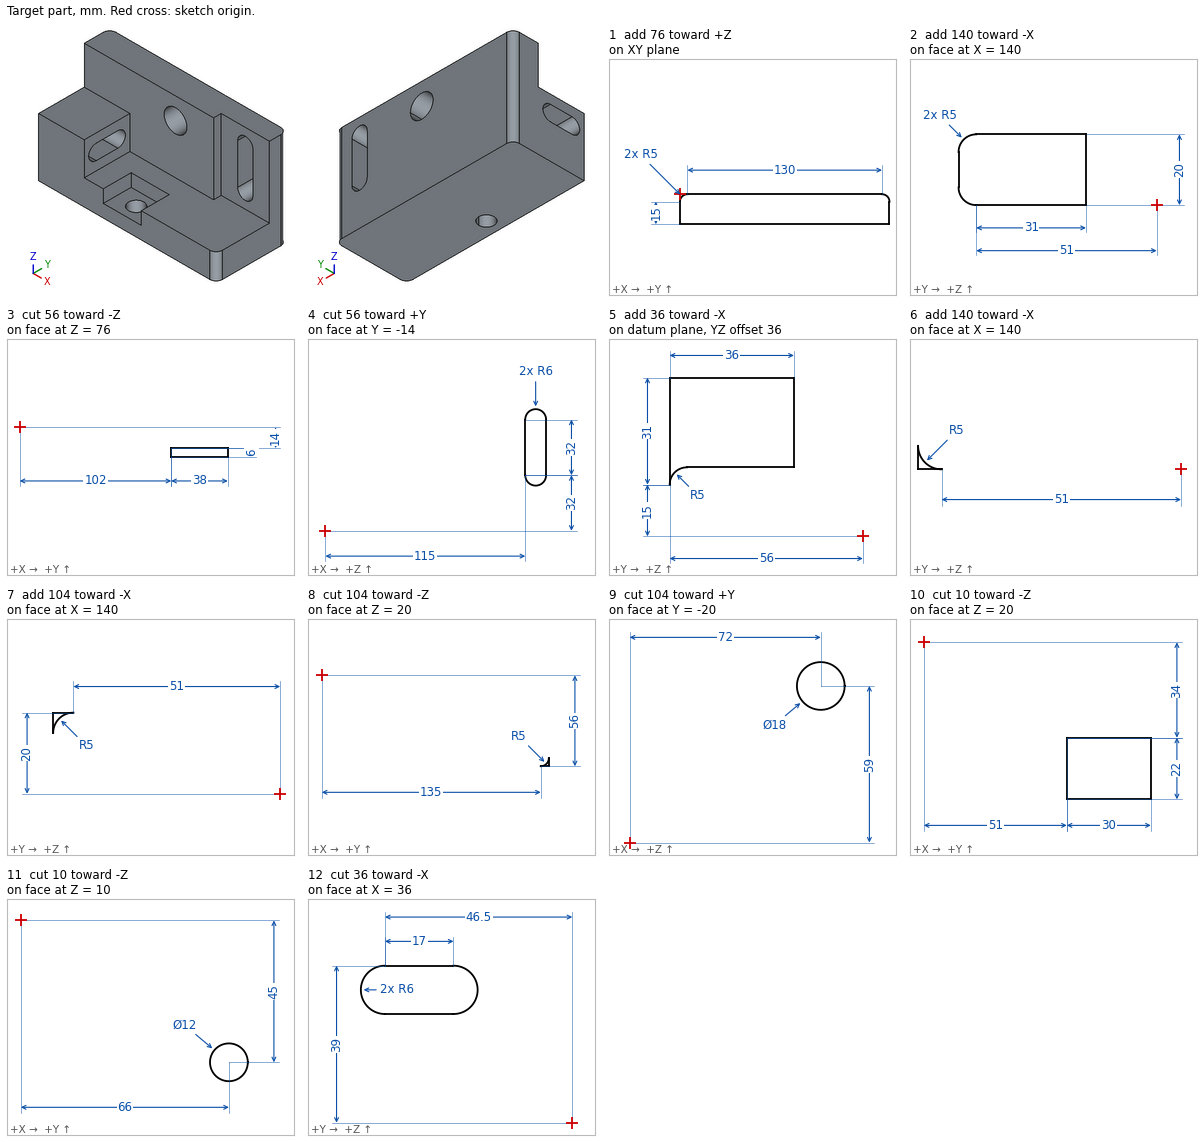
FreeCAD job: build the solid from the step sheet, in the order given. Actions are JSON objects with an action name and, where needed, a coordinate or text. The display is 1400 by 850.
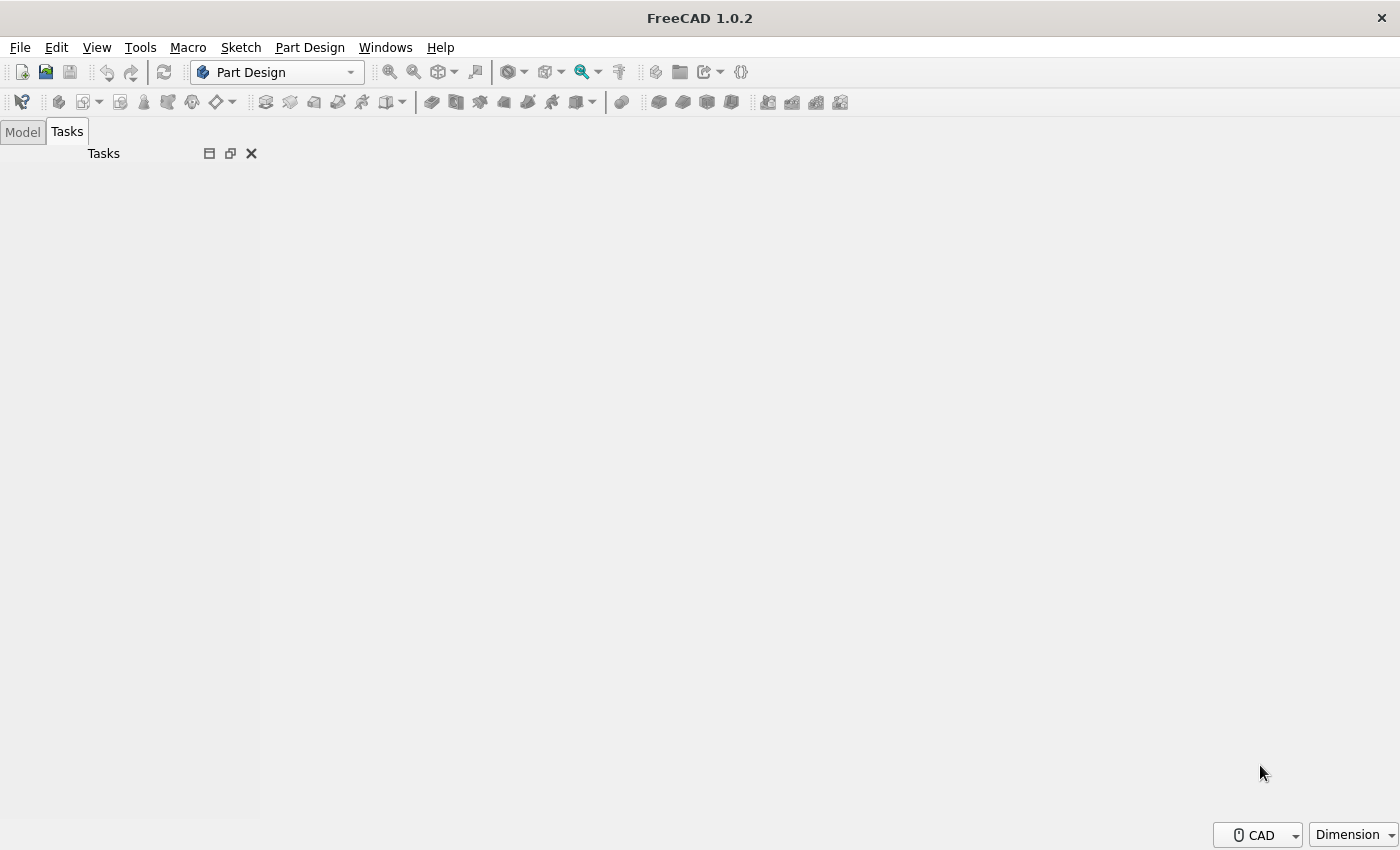
{"action": "left_click", "coordinate": [22, 72]}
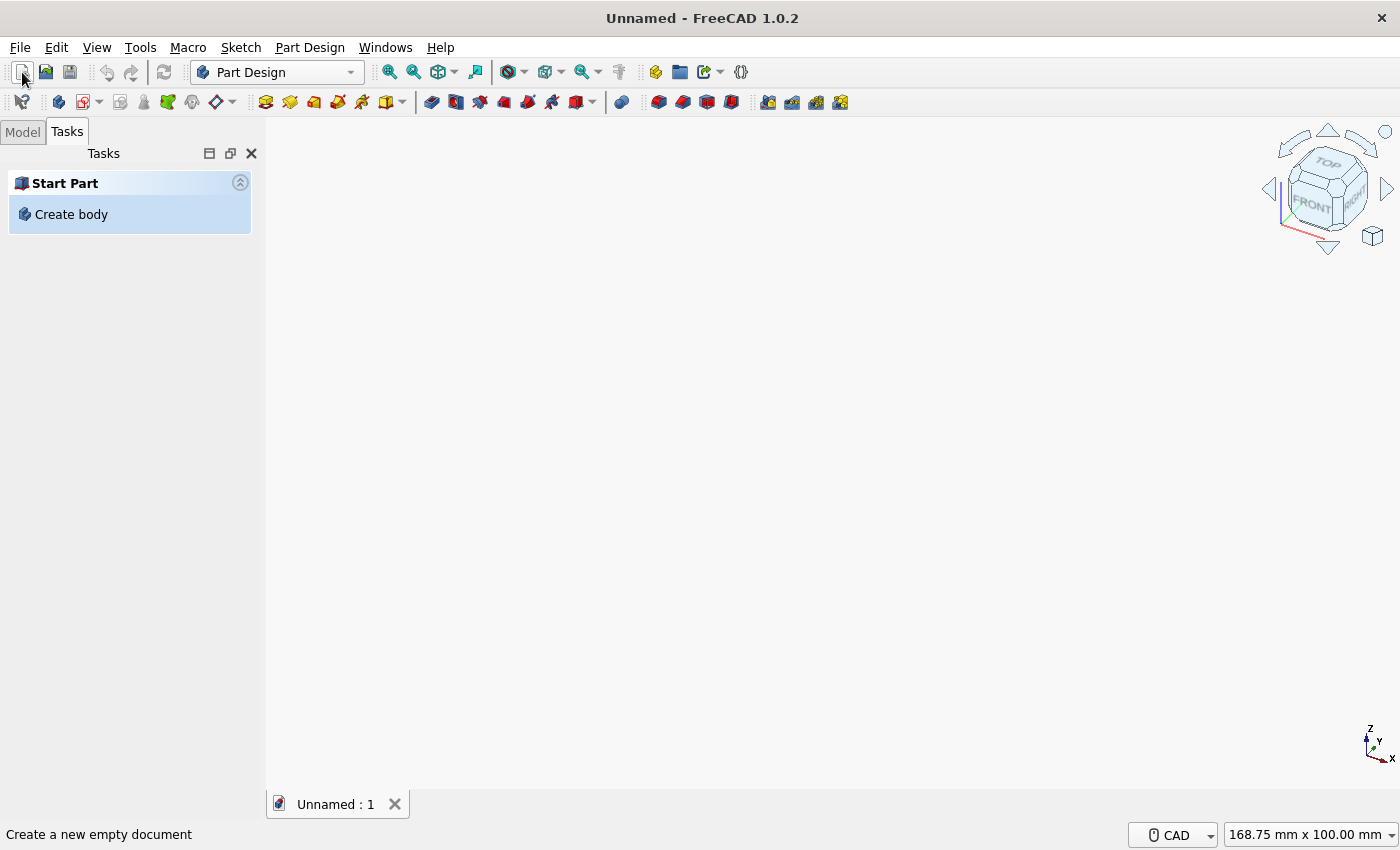
{"action": "left_click", "coordinate": [84, 102]}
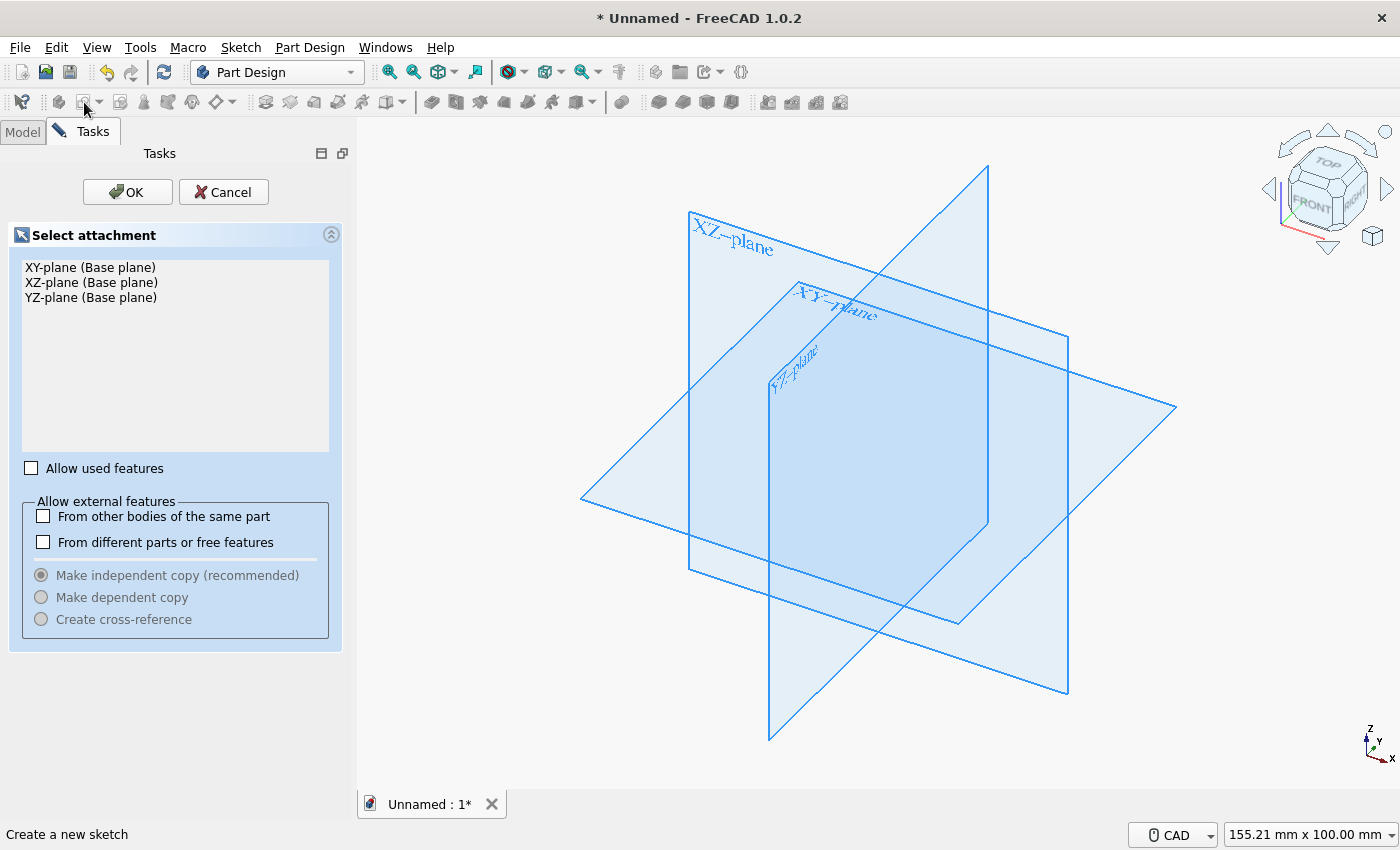
{"action": "left_click", "coordinate": [82, 268]}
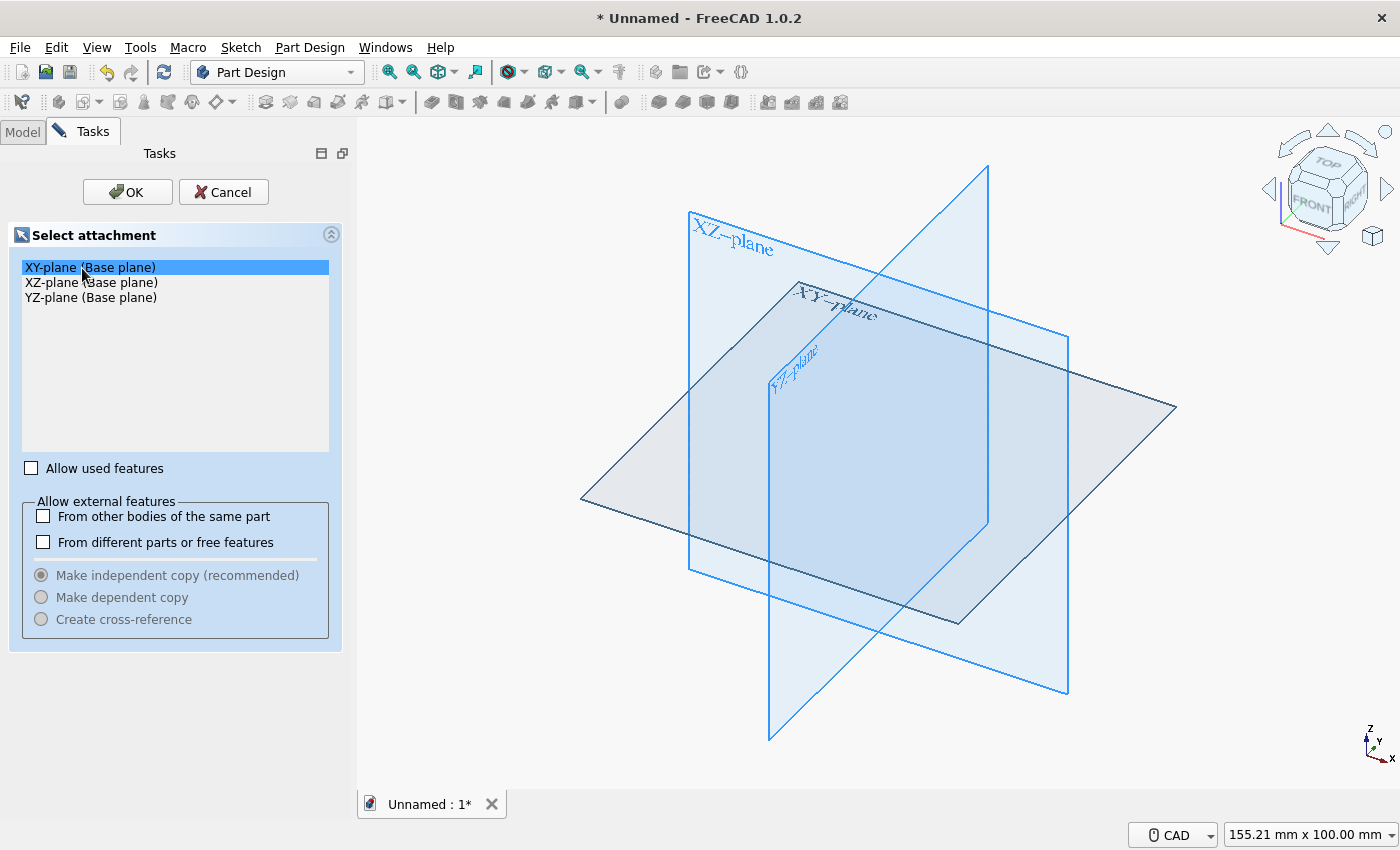
{"action": "left_click", "coordinate": [128, 192]}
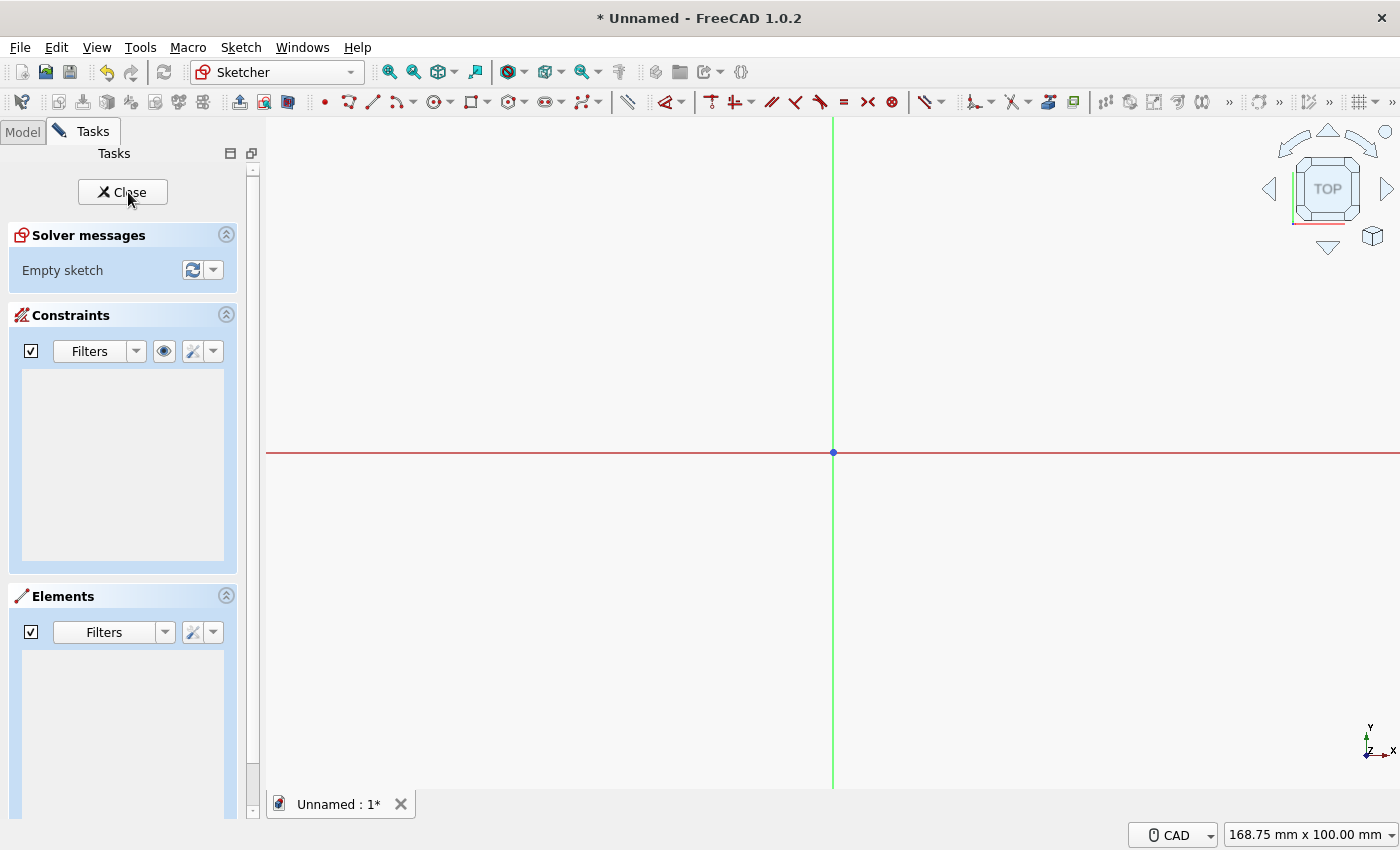
{"action": "scroll", "coordinate": [294, 371], "scroll_direction": "down", "scroll_amount": 3}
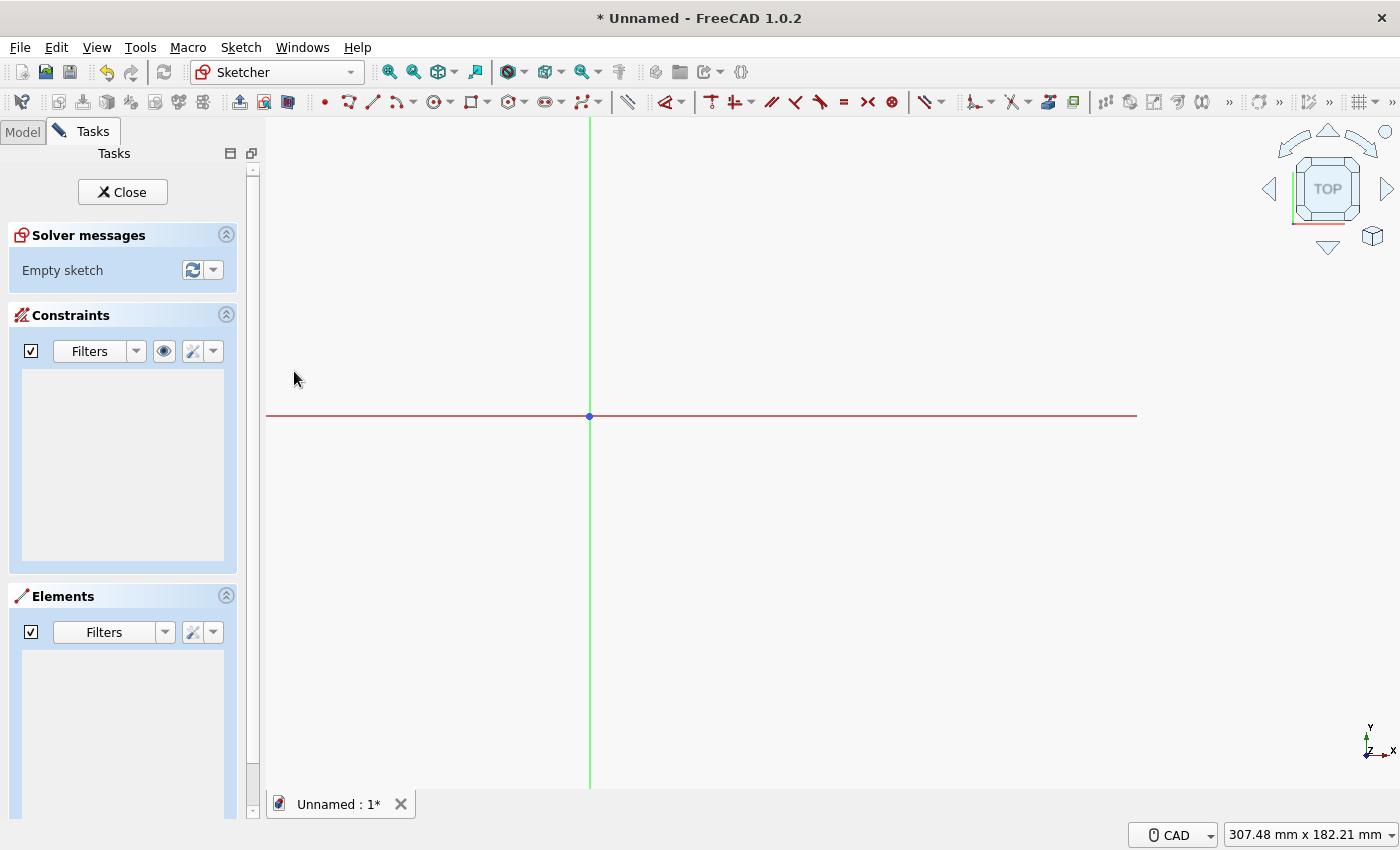
{"action": "left_click", "coordinate": [374, 102]}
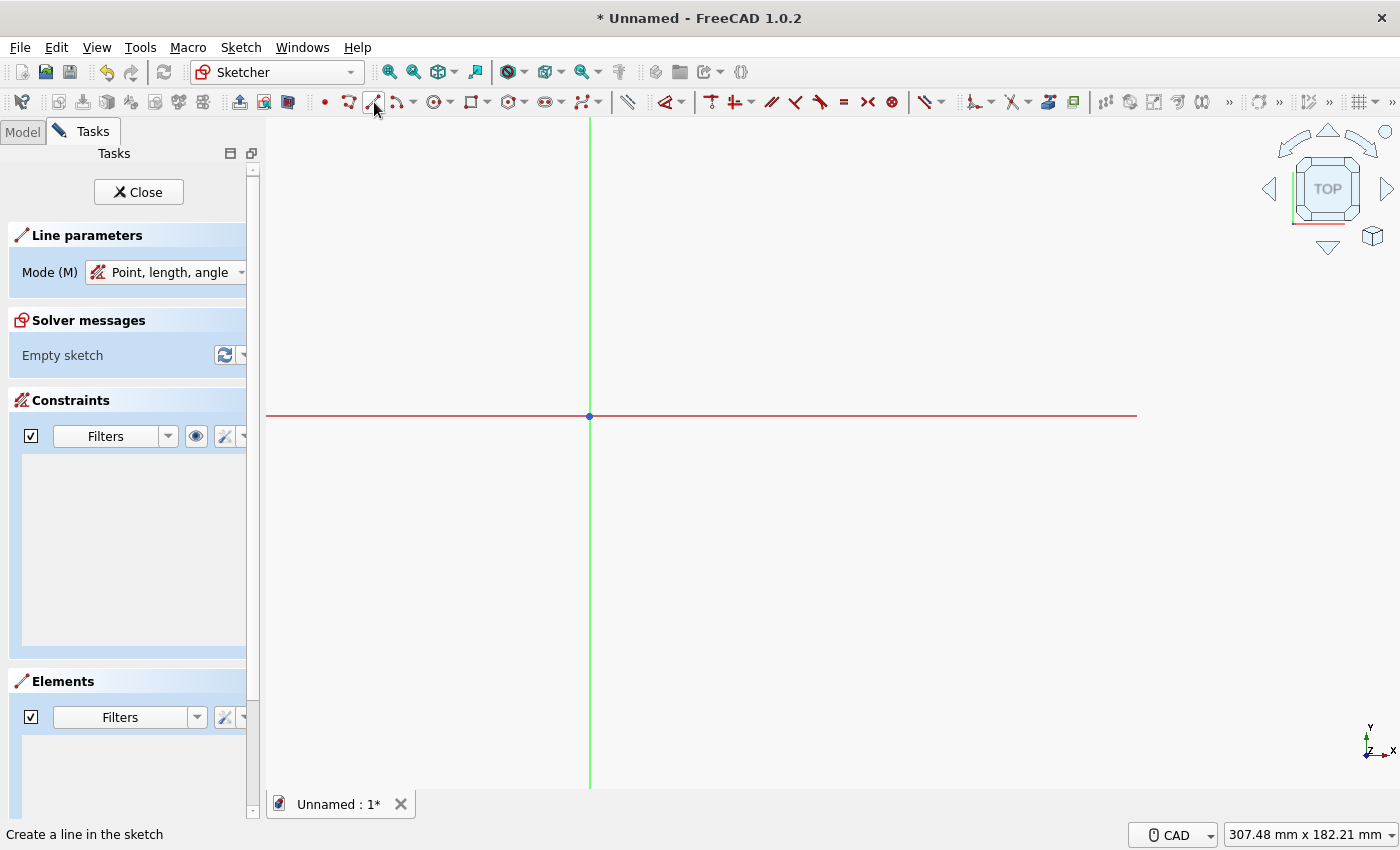
{"action": "left_click", "coordinate": [1088, 416]}
{"action": "left_click", "coordinate": [608, 425]}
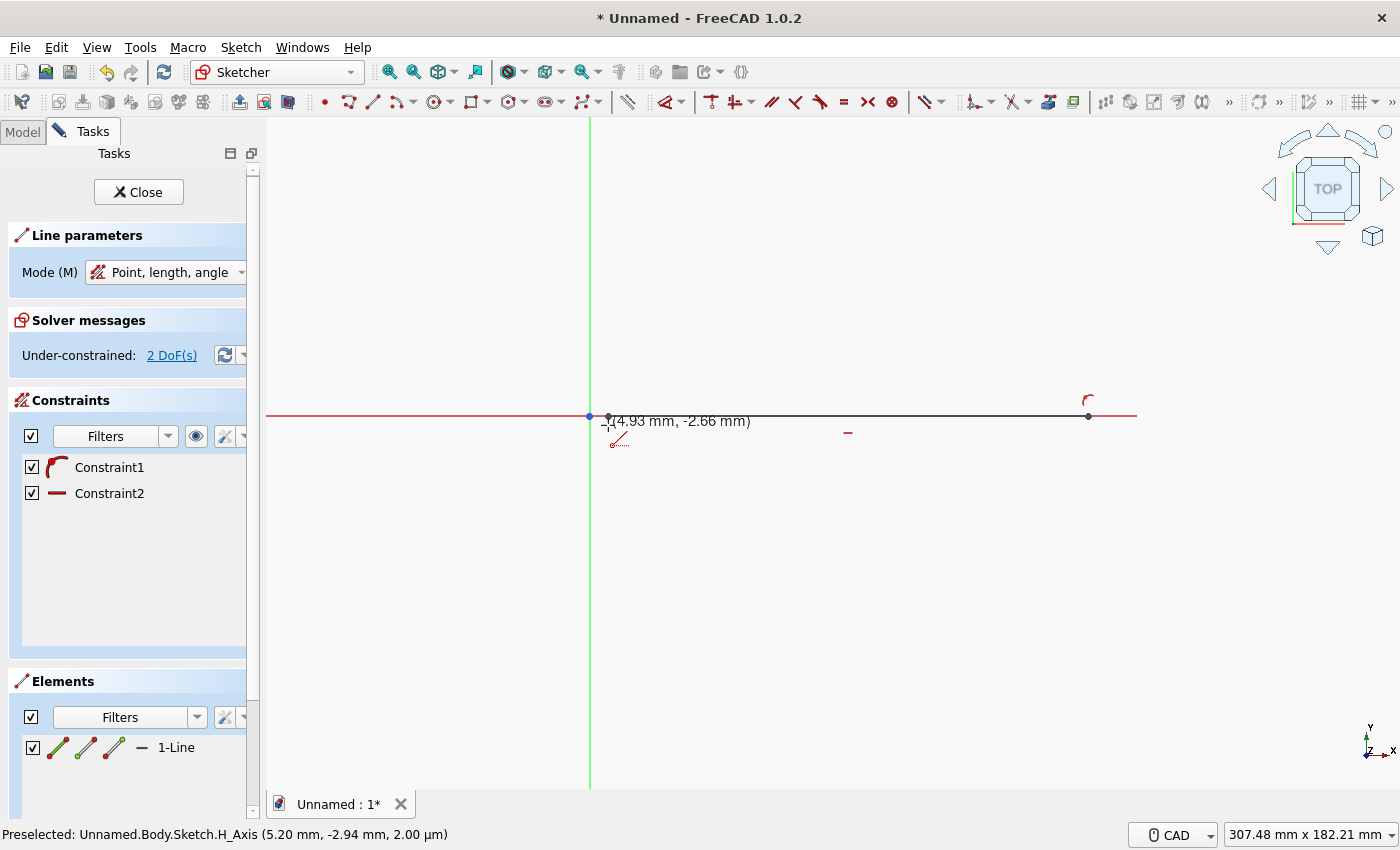
{"action": "left_click", "coordinate": [350, 102]}